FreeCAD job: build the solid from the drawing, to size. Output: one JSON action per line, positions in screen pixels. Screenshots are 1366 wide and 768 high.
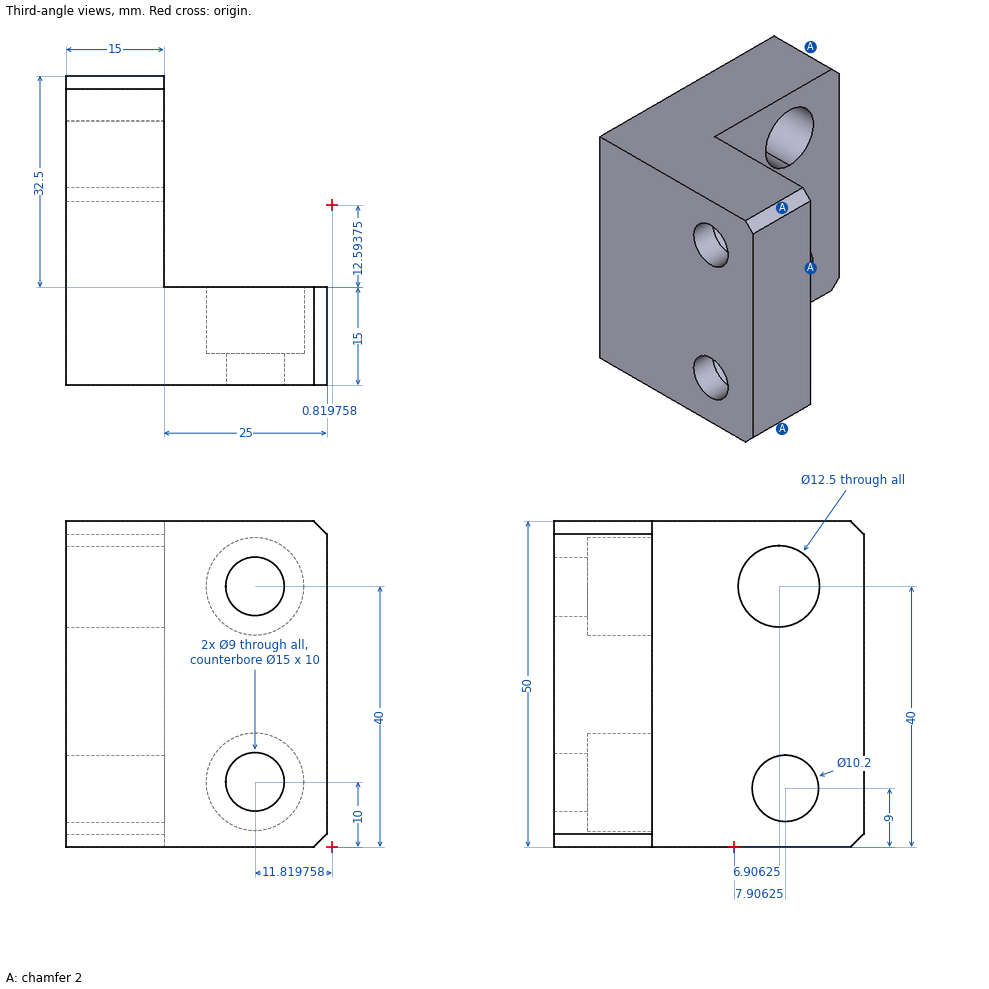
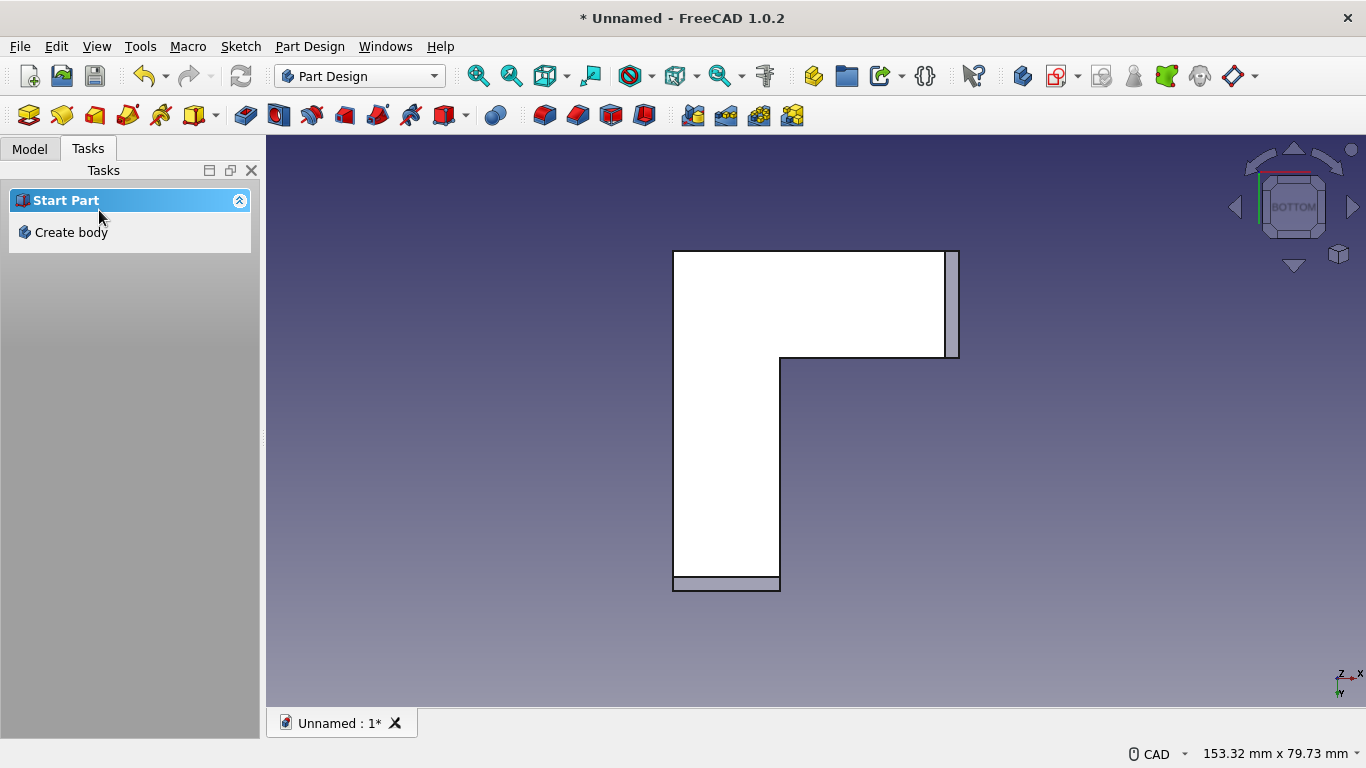
{"action": "key", "text": "4"}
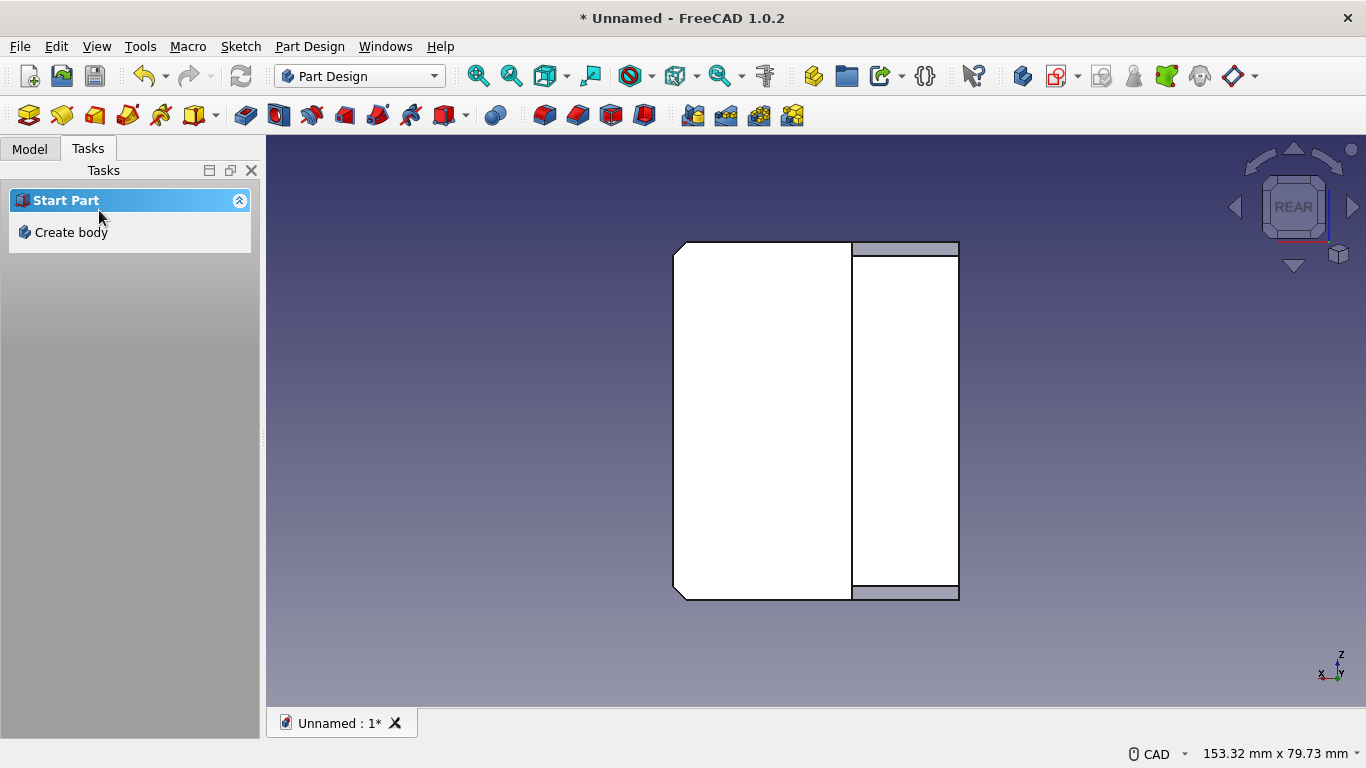
{"action": "left_click", "coordinate": [762, 369]}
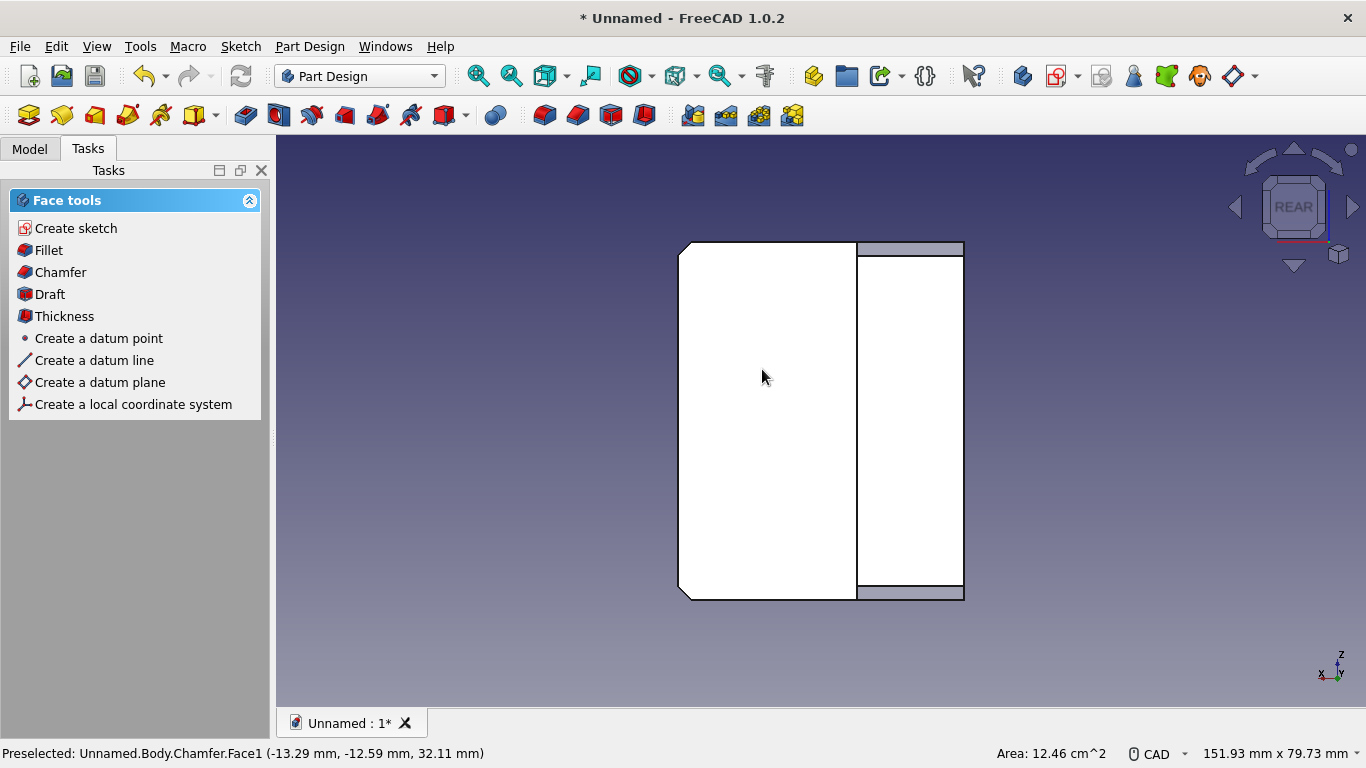
{"action": "left_click", "coordinate": [1056, 76]}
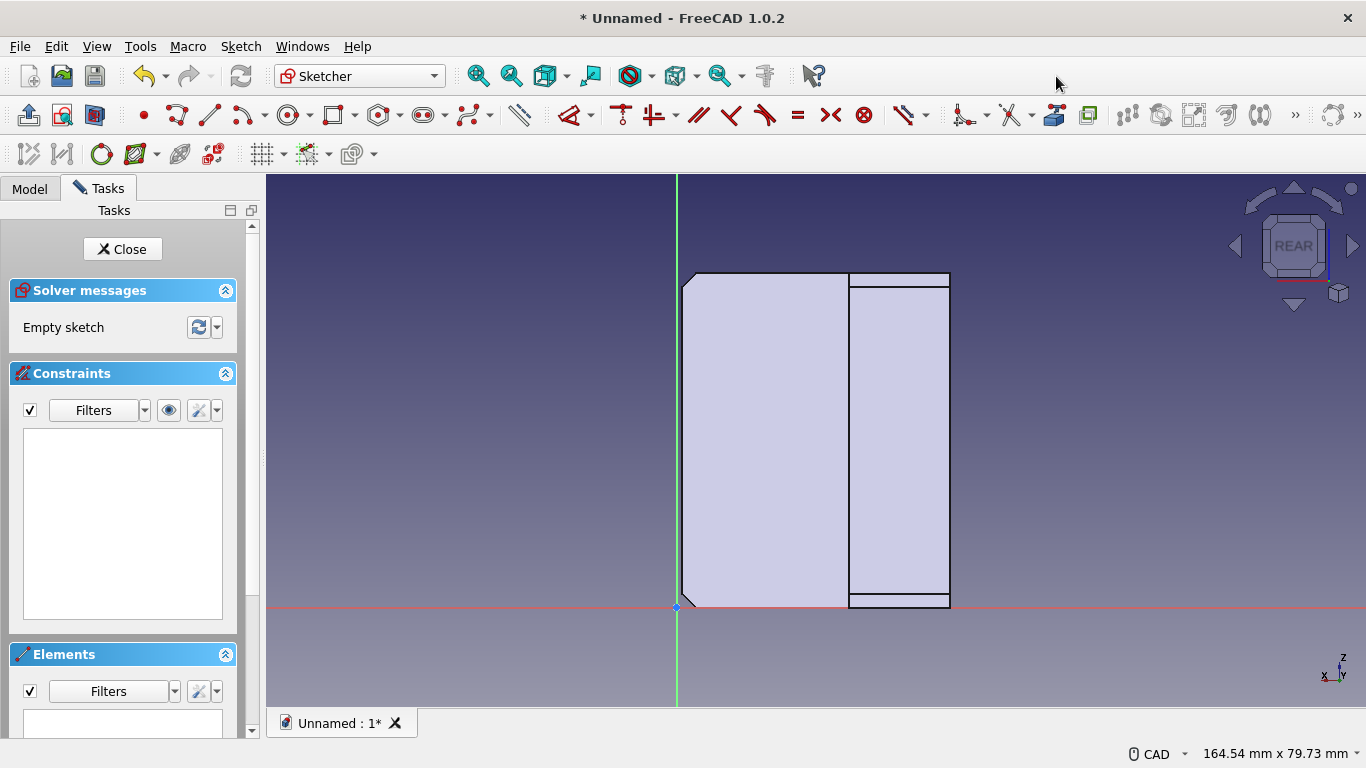
{"action": "left_click", "coordinate": [288, 116]}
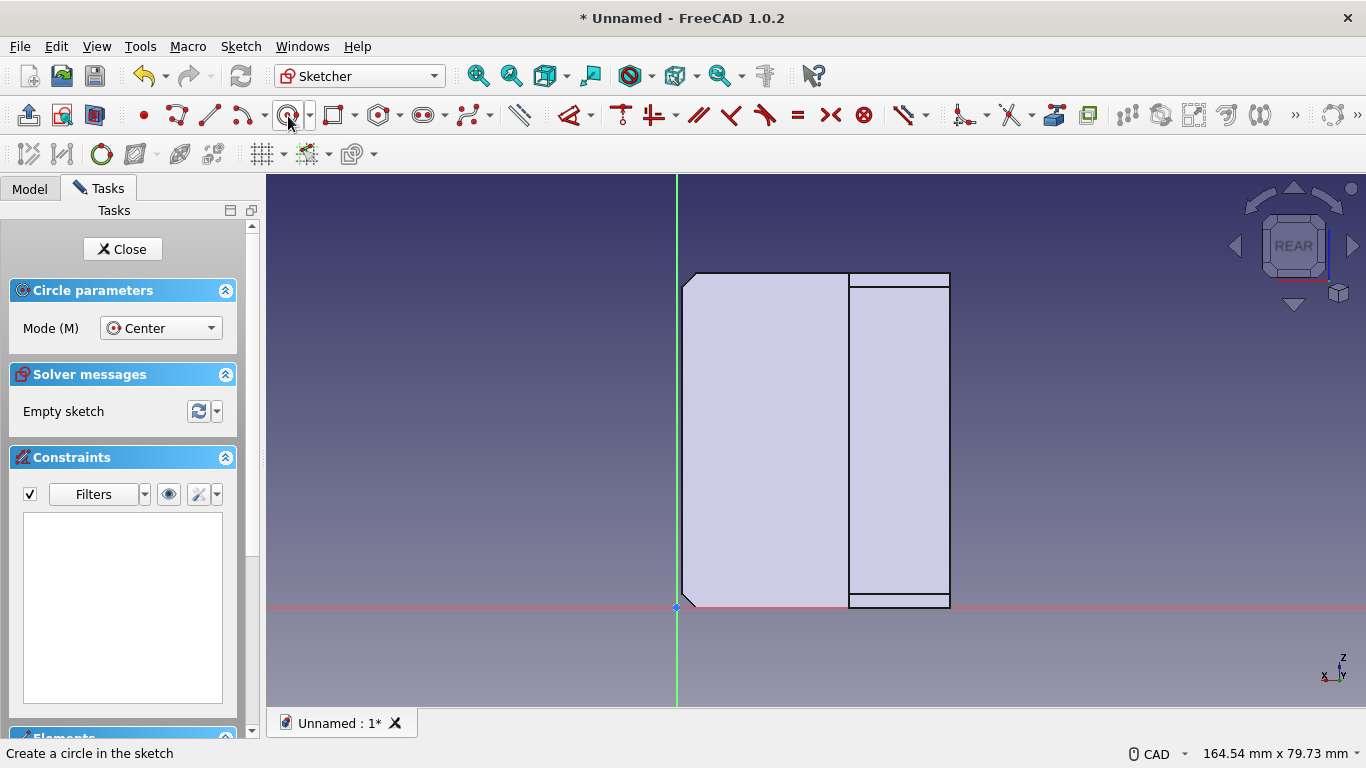
{"action": "left_click", "coordinate": [756, 541]}
{"action": "left_click", "coordinate": [777, 520]}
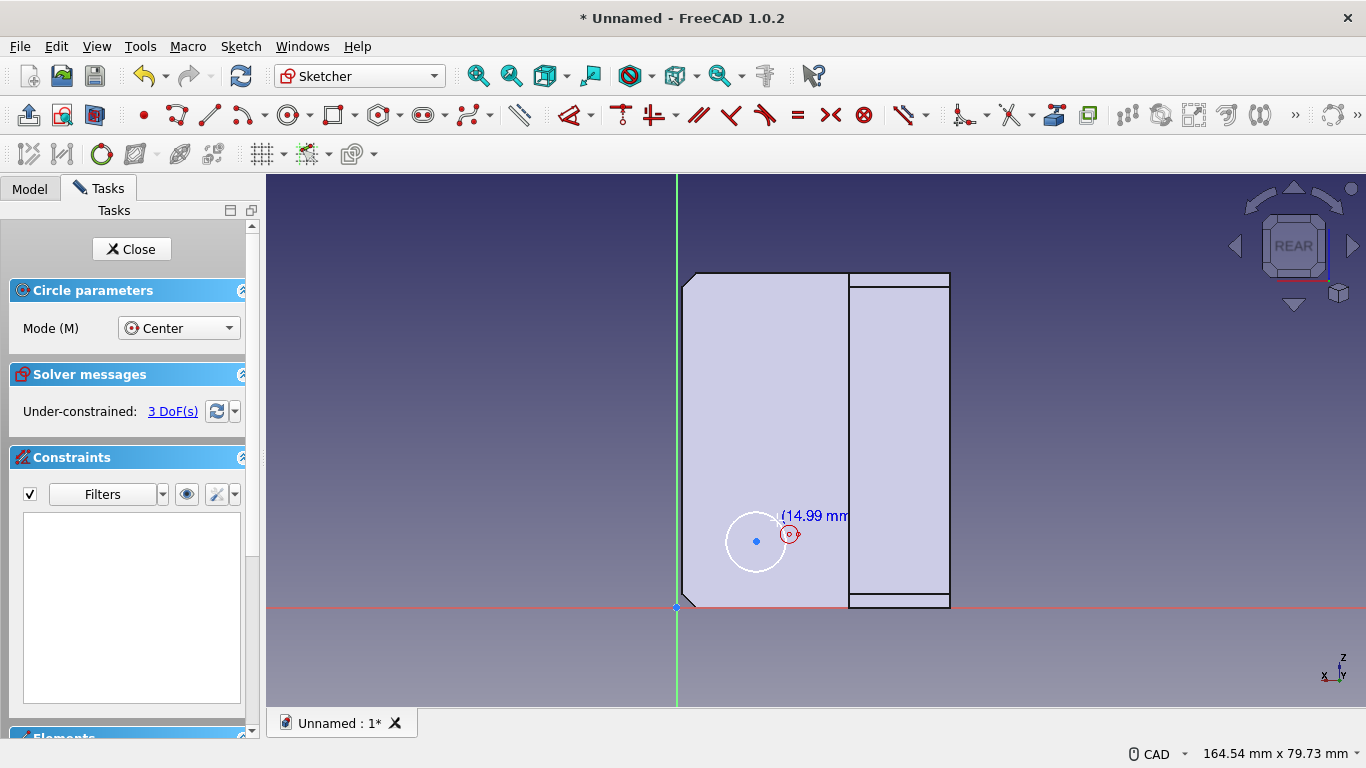
{"action": "left_click", "coordinate": [756, 340]}
{"action": "left_click", "coordinate": [777, 319]}
{"action": "key", "text": "Escape"}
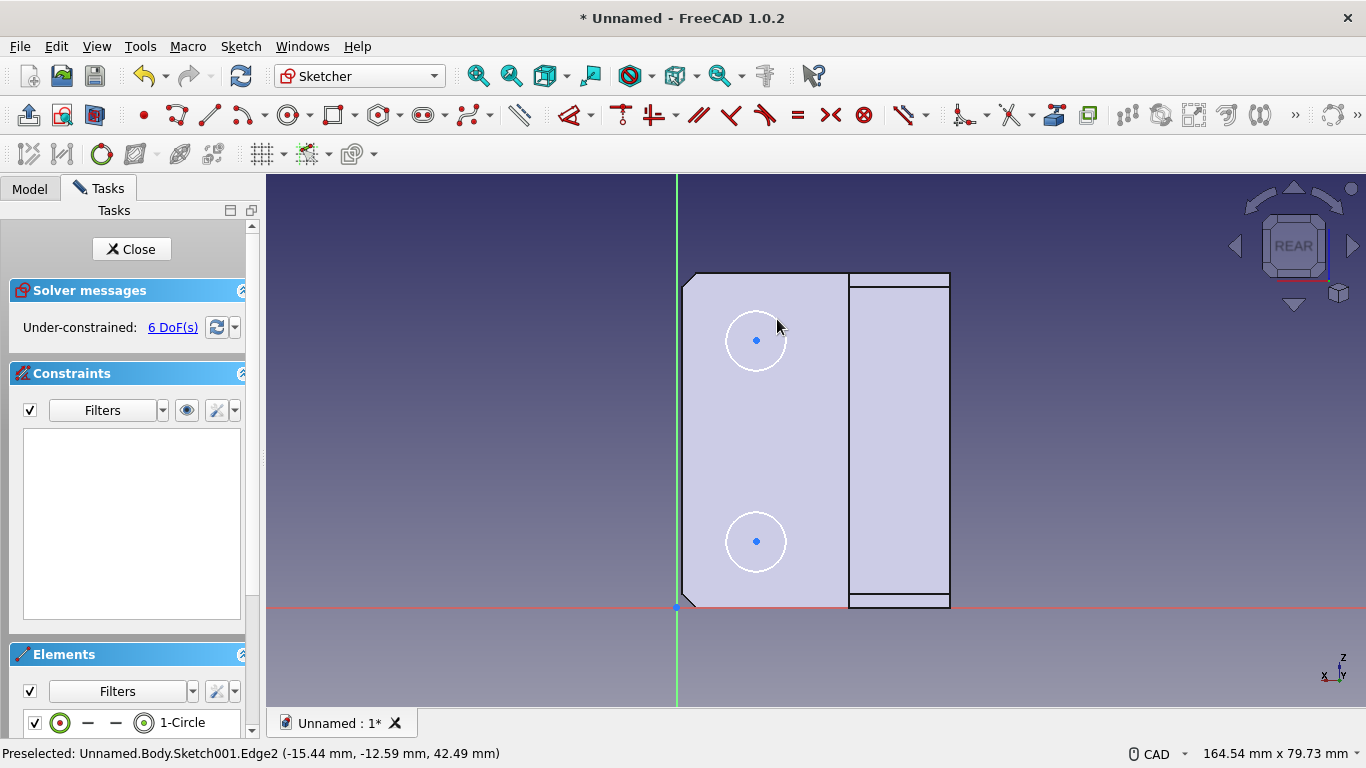
{"action": "left_click", "coordinate": [777, 521]}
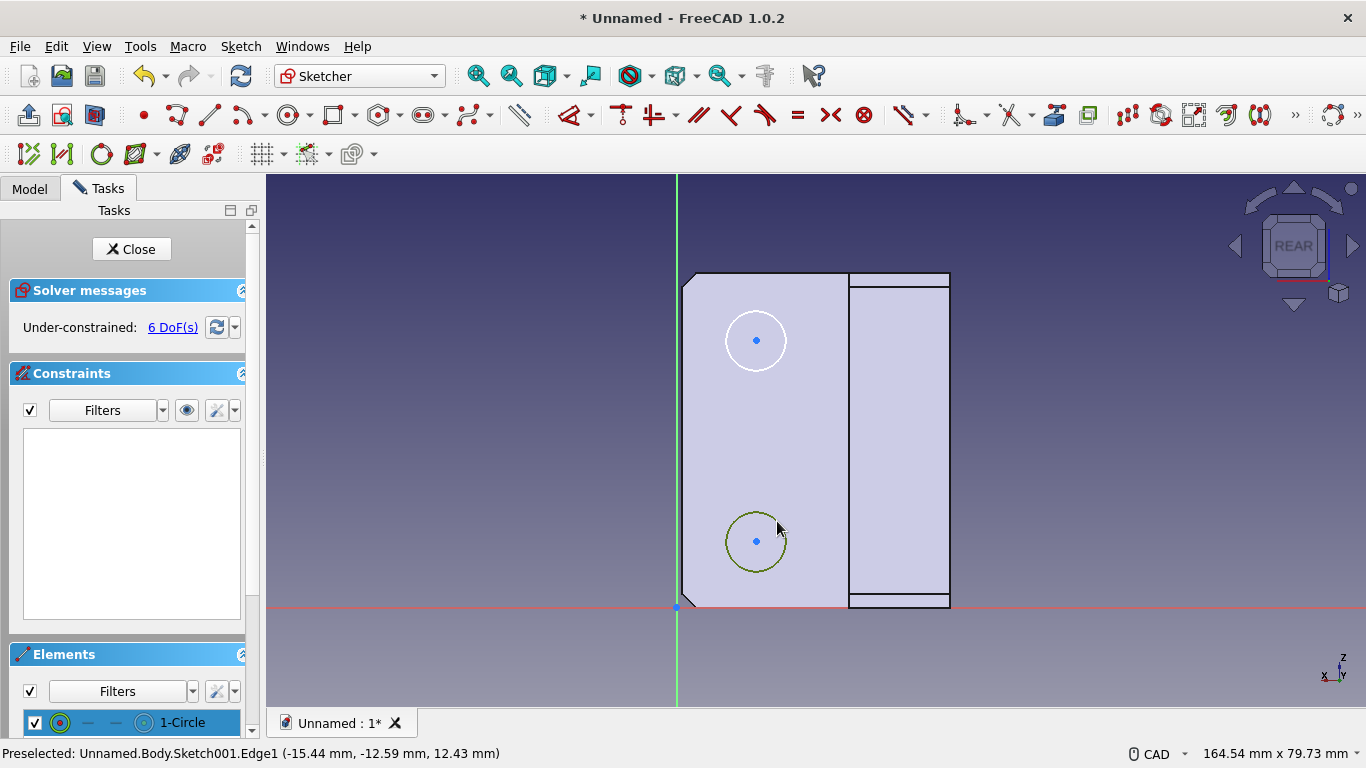
{"action": "left_click", "coordinate": [777, 320]}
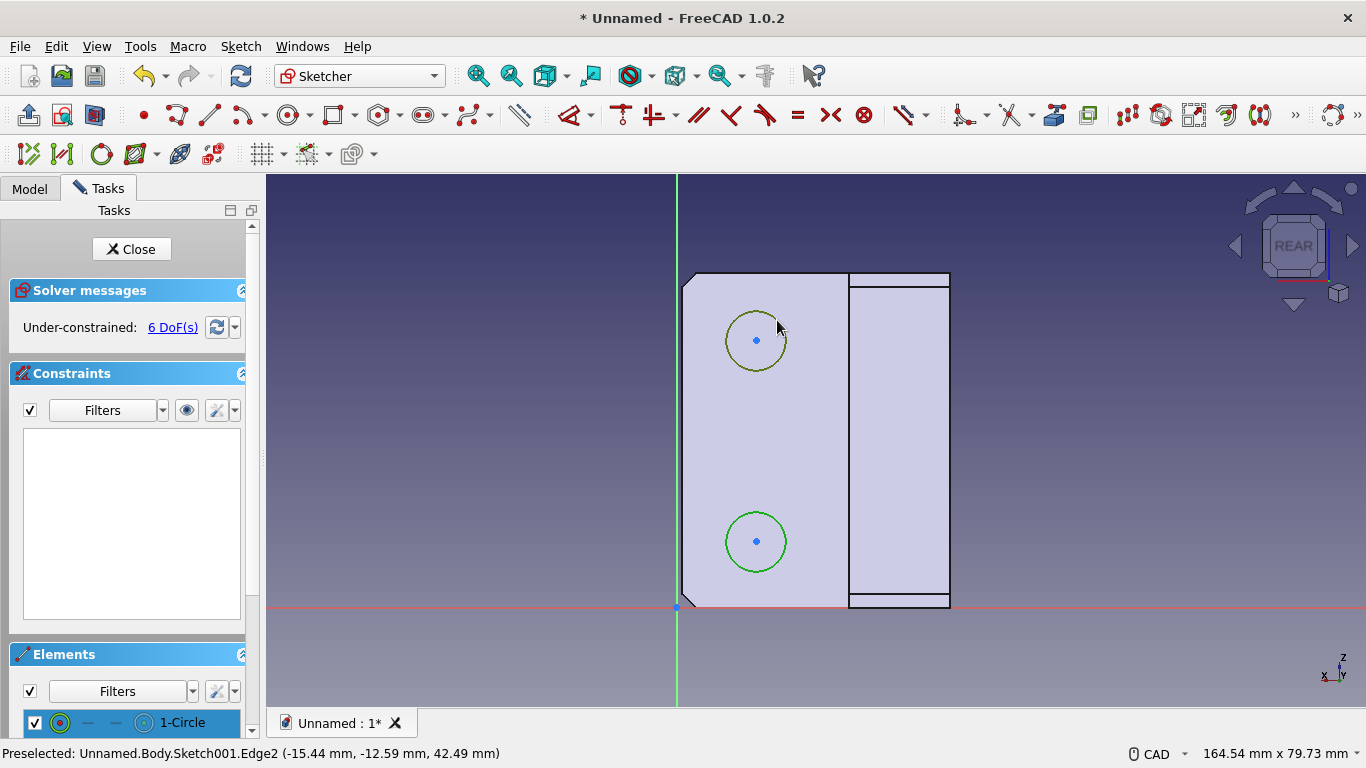
{"action": "left_click", "coordinate": [798, 116]}